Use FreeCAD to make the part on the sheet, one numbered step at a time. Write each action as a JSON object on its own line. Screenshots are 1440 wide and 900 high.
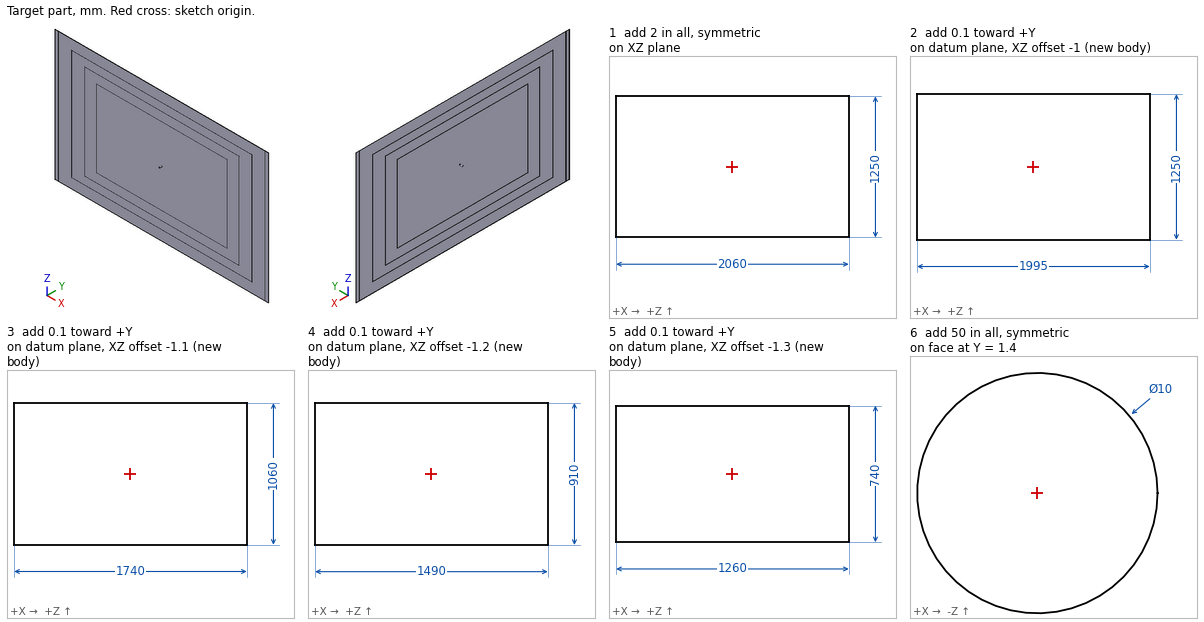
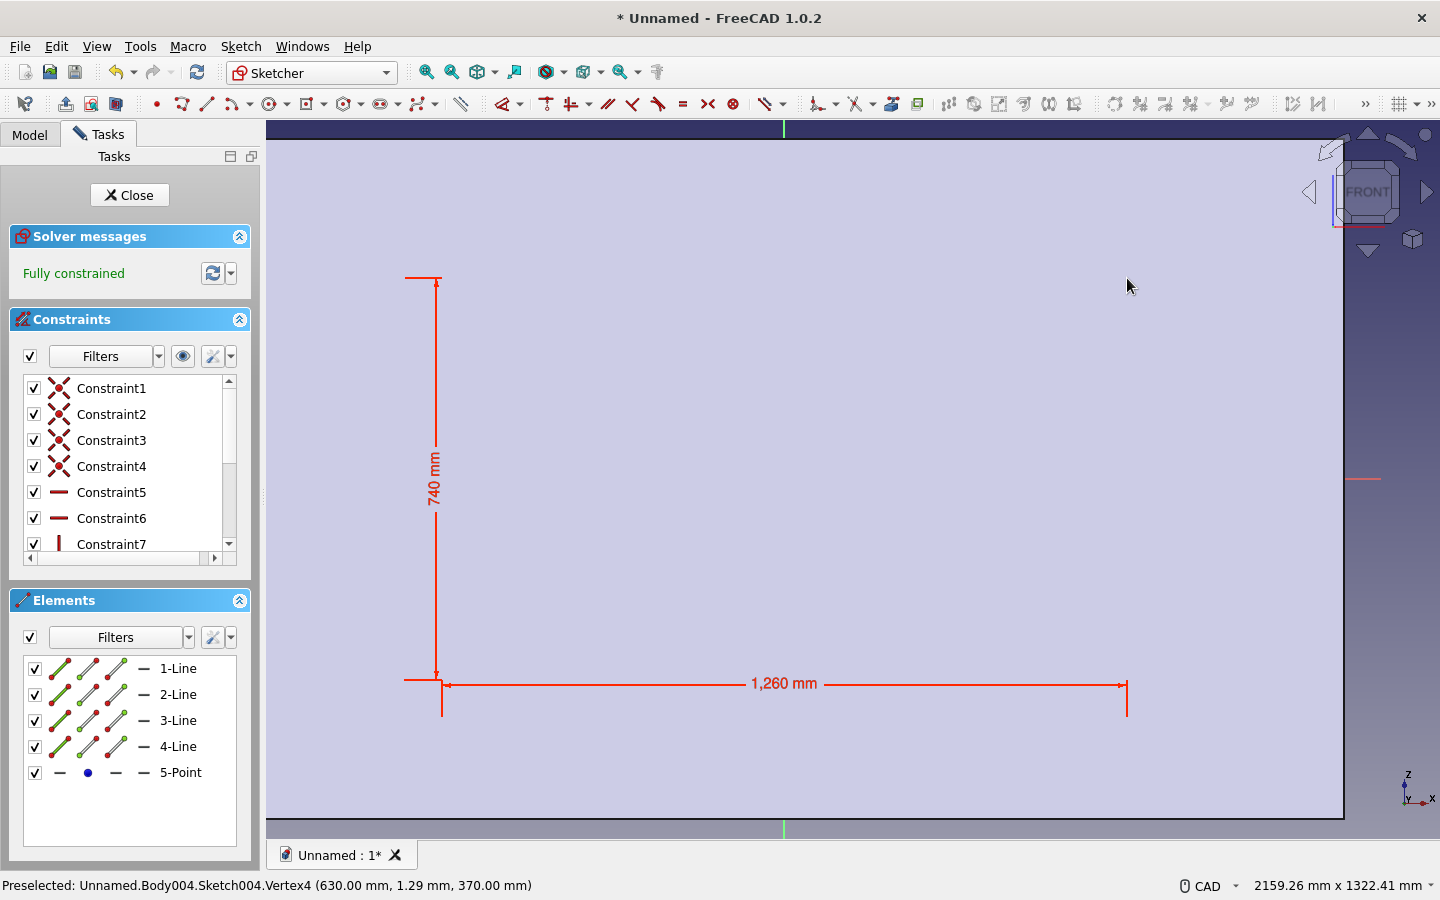
{"action": "left_click", "coordinate": [130, 195]}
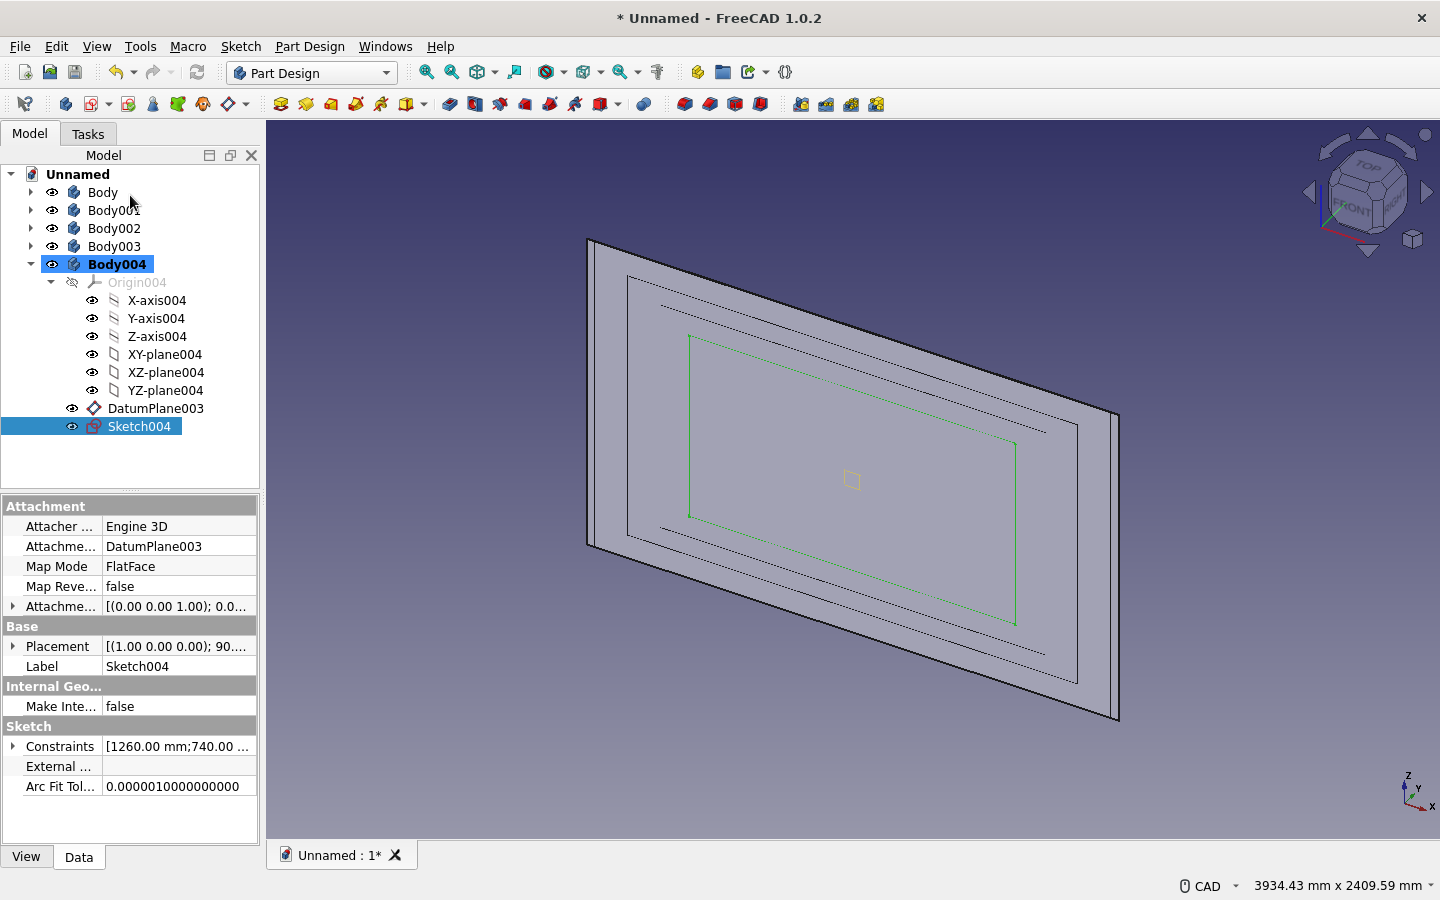
{"action": "left_click", "coordinate": [281, 104]}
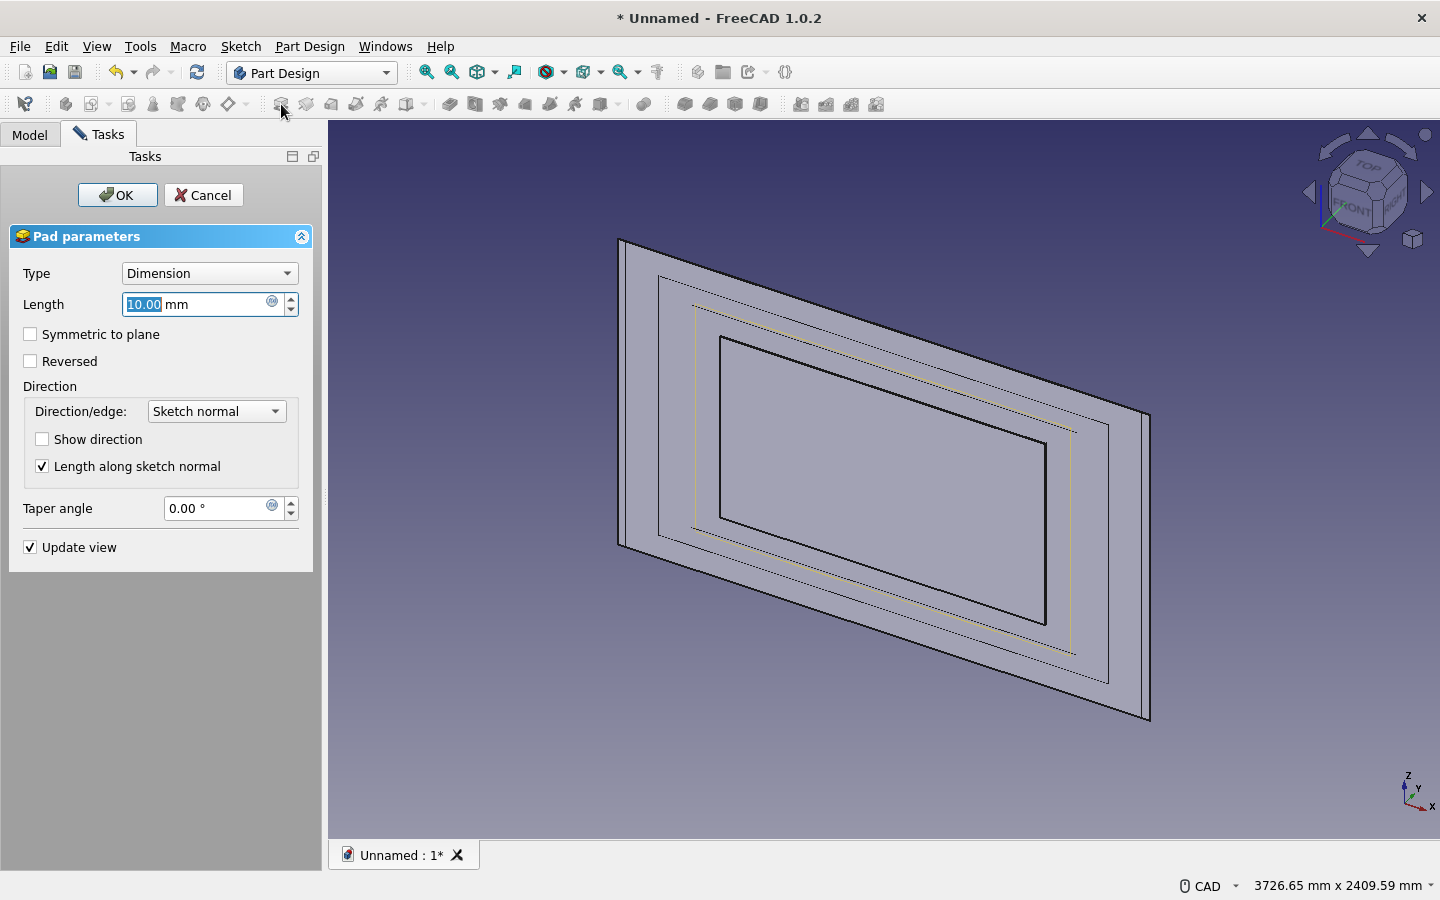
{"action": "type", "text": "0.1"}
{"action": "key", "text": "Tab"}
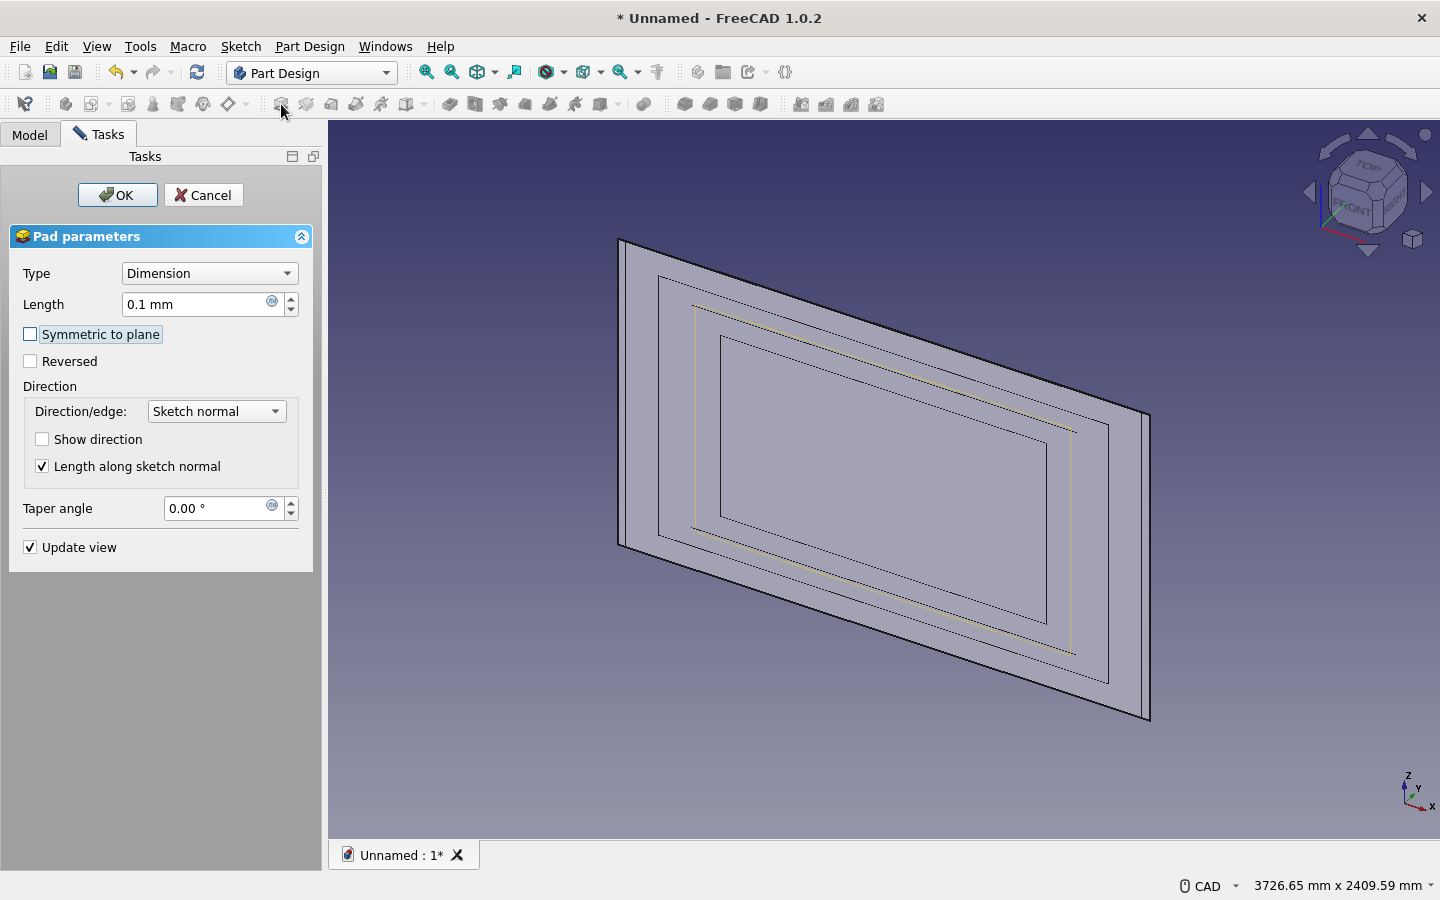
{"action": "left_click", "coordinate": [31, 361]}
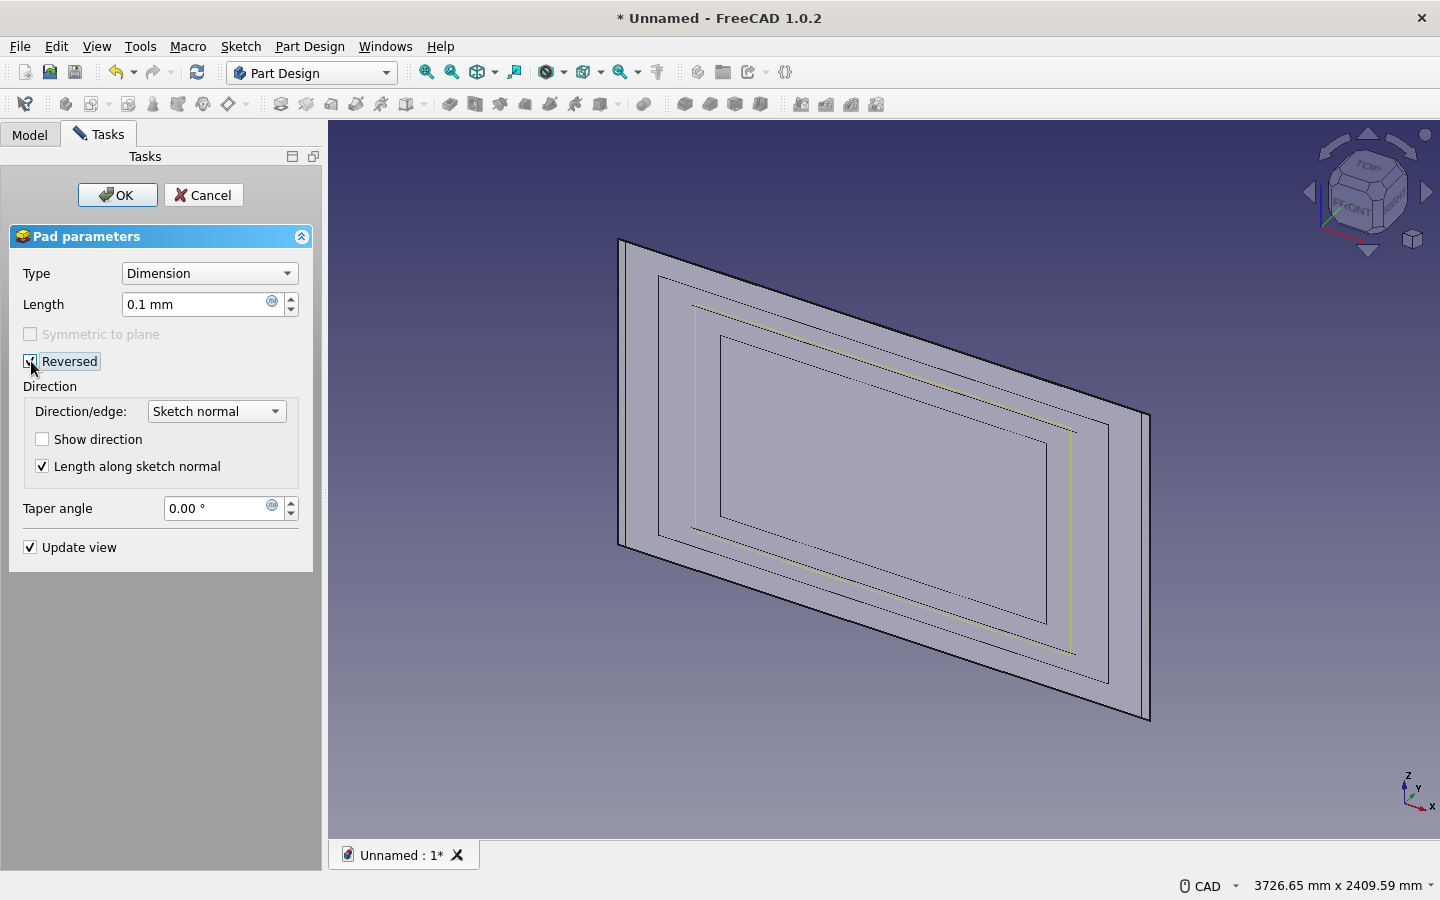
{"action": "left_click", "coordinate": [118, 195]}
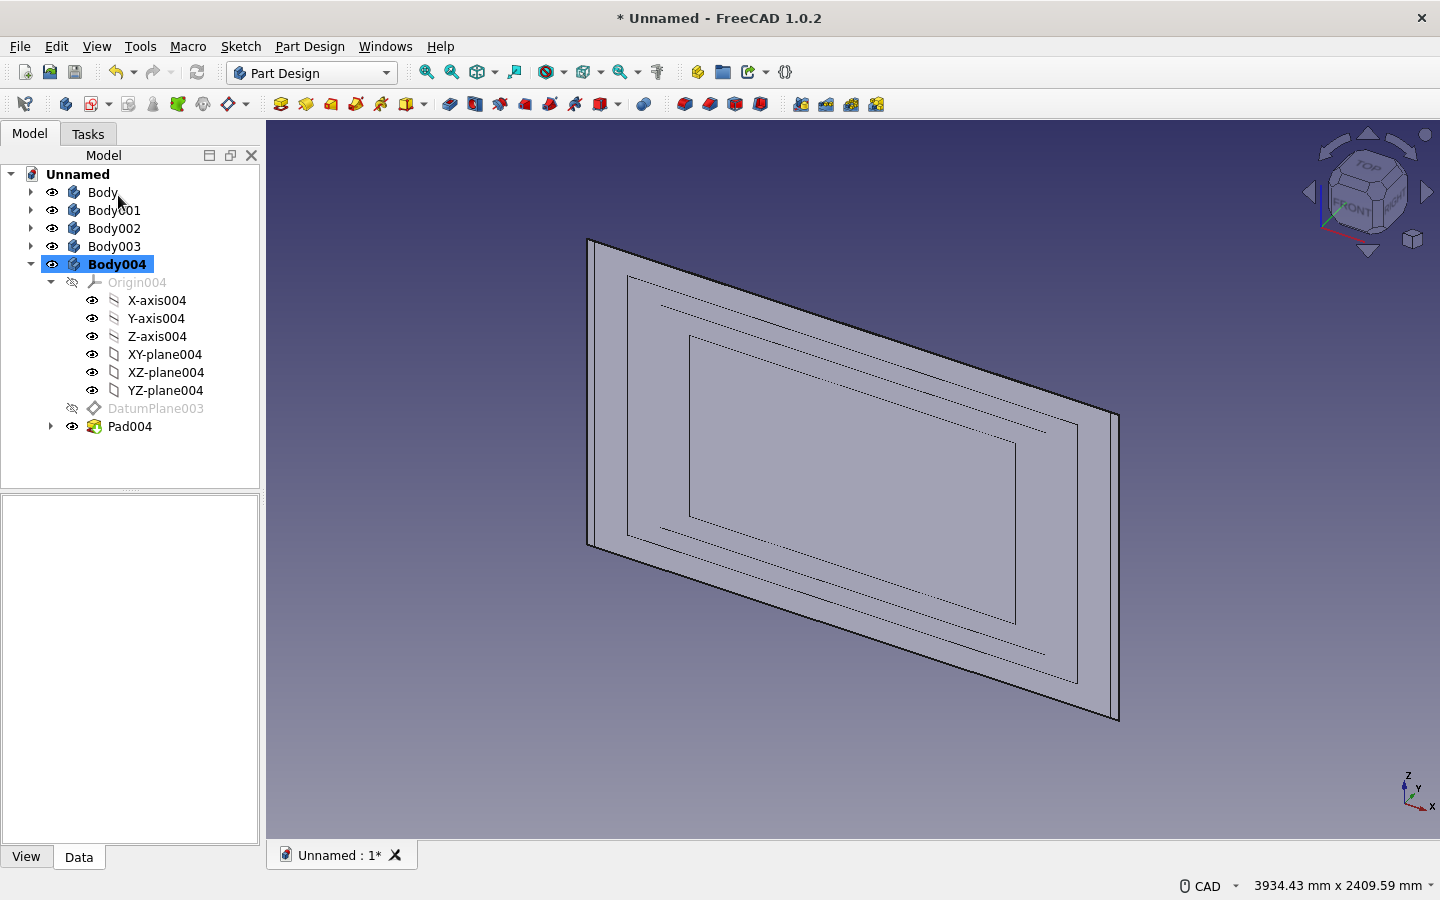
{"action": "left_click", "coordinate": [427, 72]}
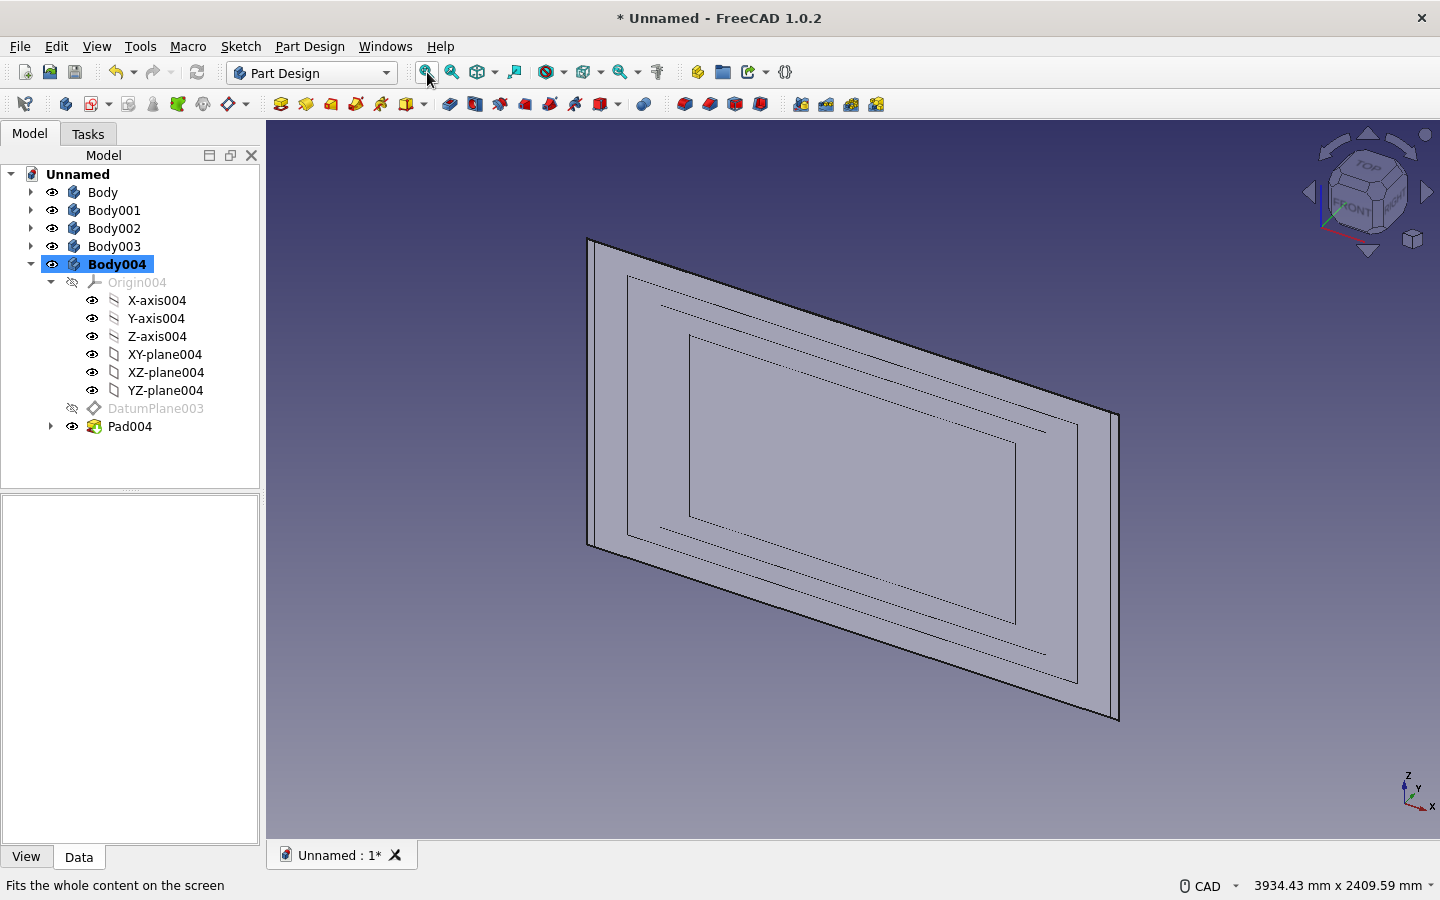
{"action": "key", "text": "4"}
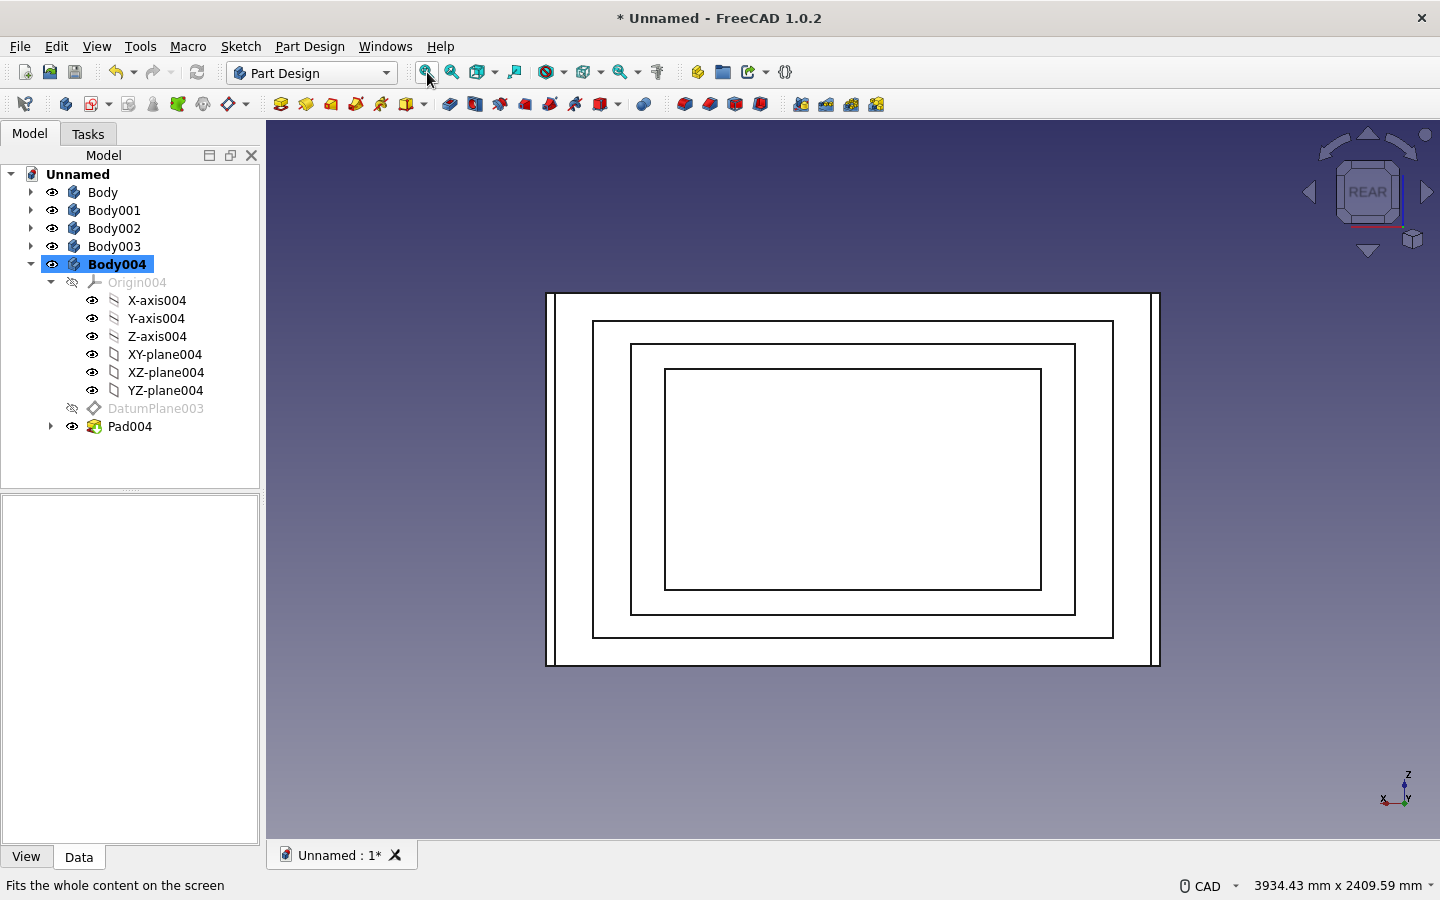
{"action": "left_click", "coordinate": [427, 72]}